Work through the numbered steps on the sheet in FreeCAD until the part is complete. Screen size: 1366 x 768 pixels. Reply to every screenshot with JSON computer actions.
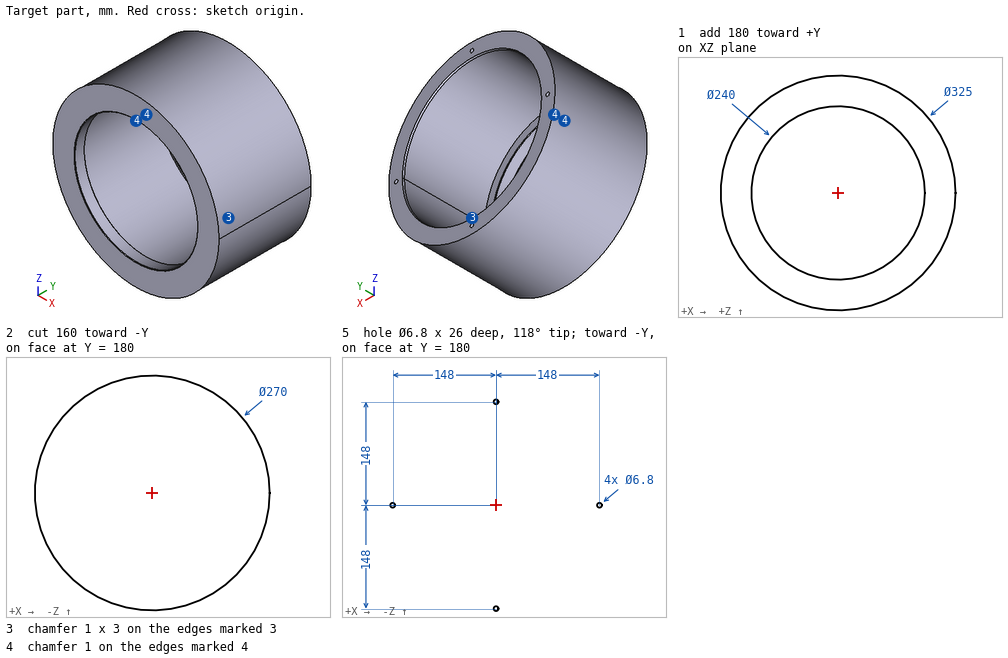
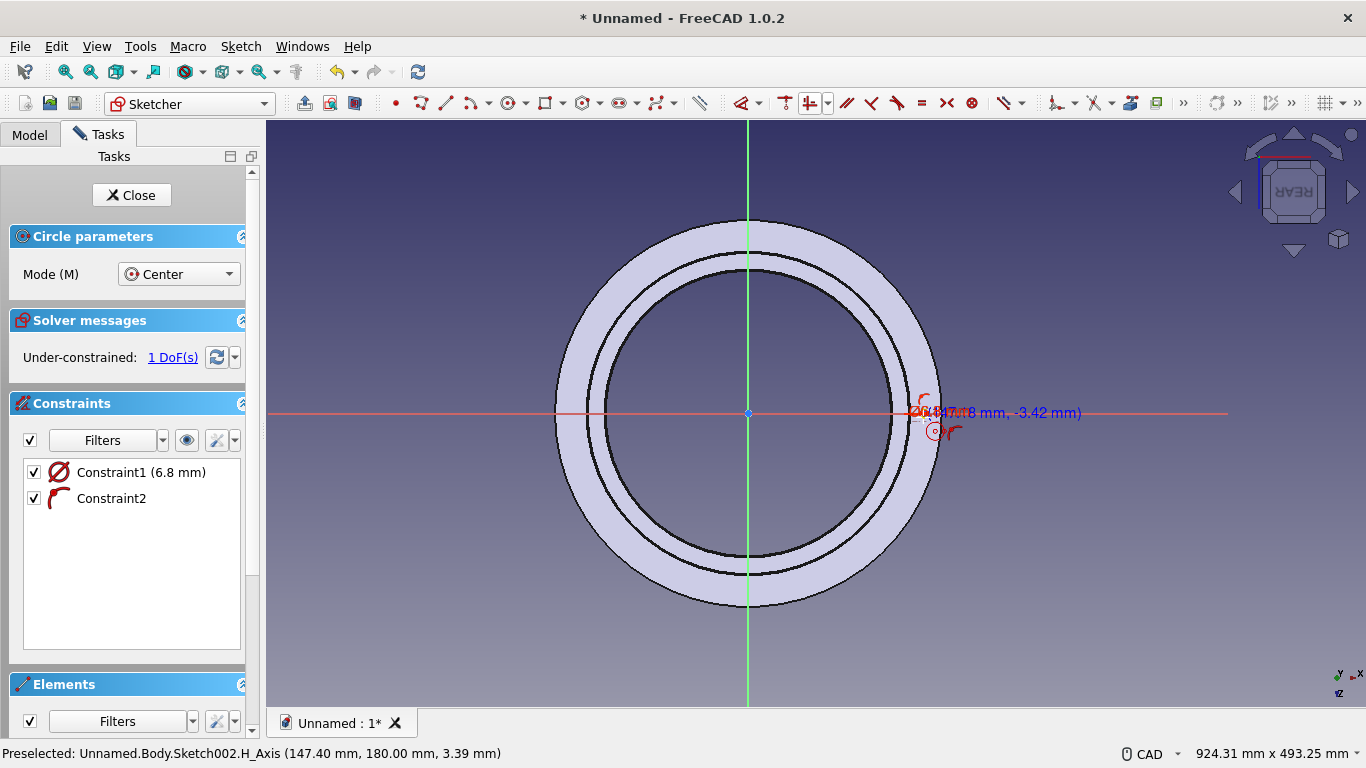
{"action": "scroll", "coordinate": [748, 590], "scroll_direction": "up", "scroll_amount": 9}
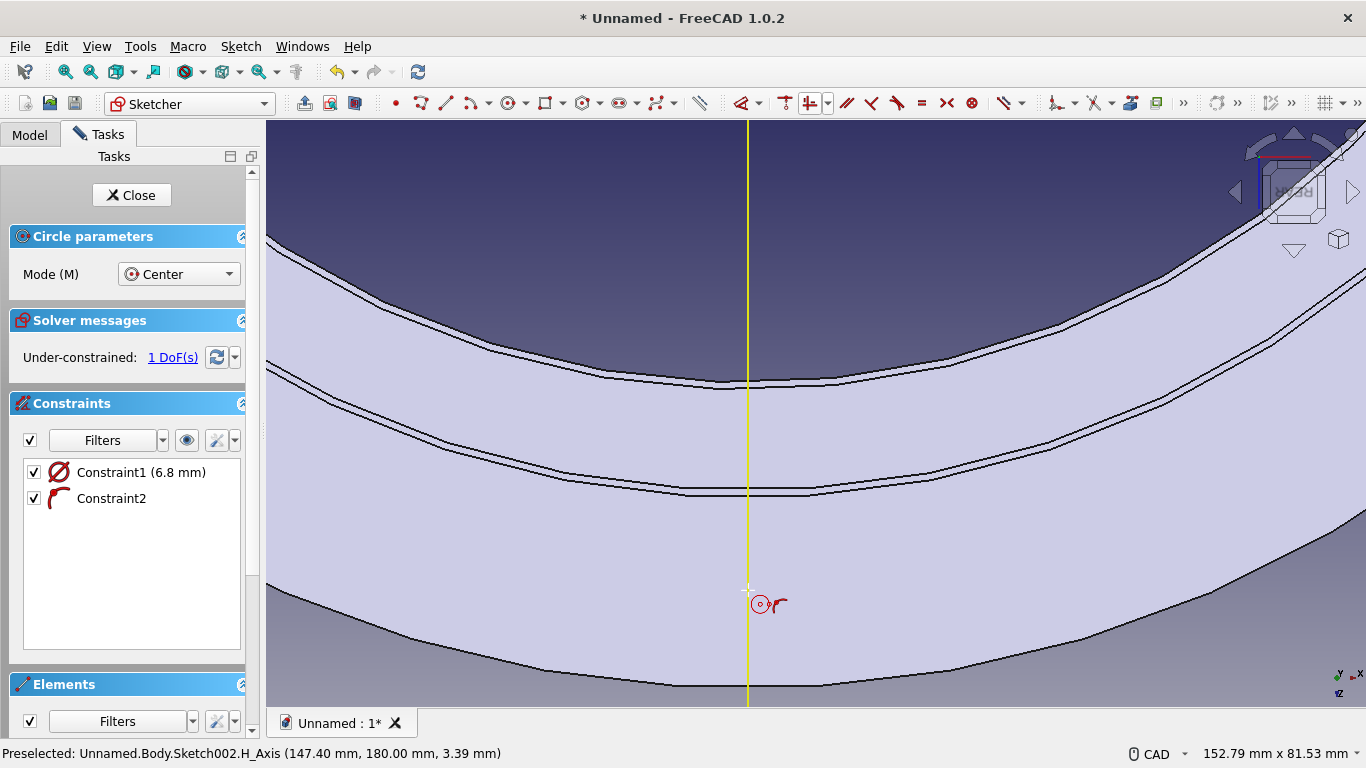
{"action": "scroll", "coordinate": [747, 591], "scroll_direction": "down", "scroll_amount": 9}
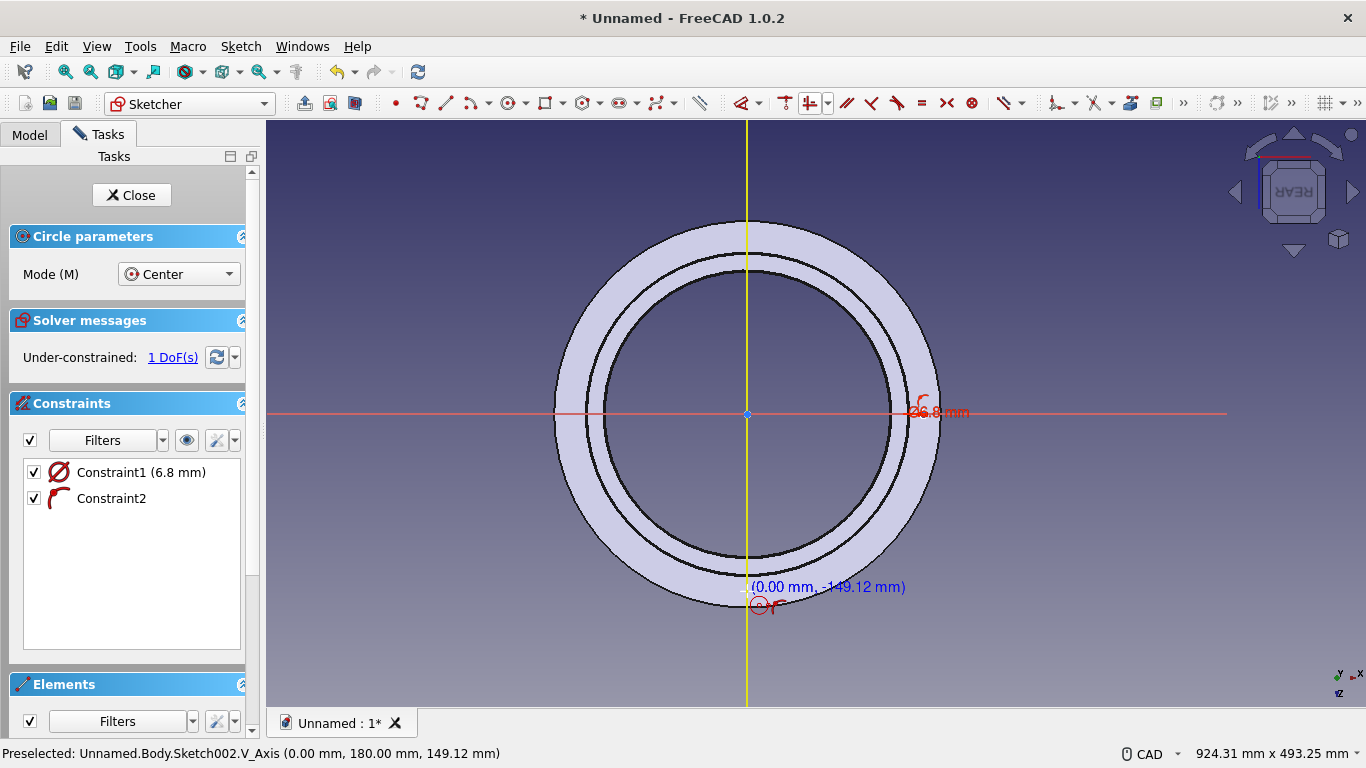
{"action": "left_click", "coordinate": [747, 591]}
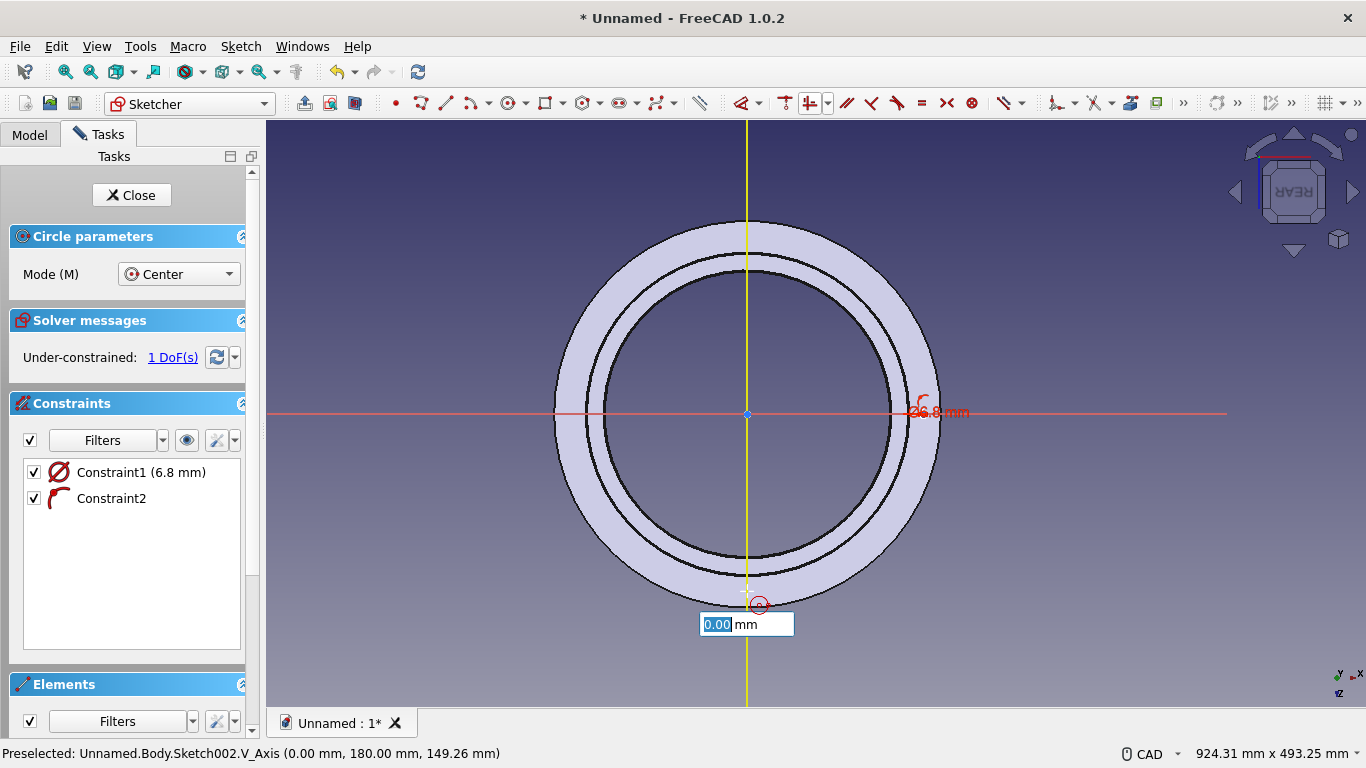
{"action": "scroll", "coordinate": [751, 589], "scroll_direction": "up", "scroll_amount": 8}
{"action": "mouse_move", "coordinate": [751, 586]}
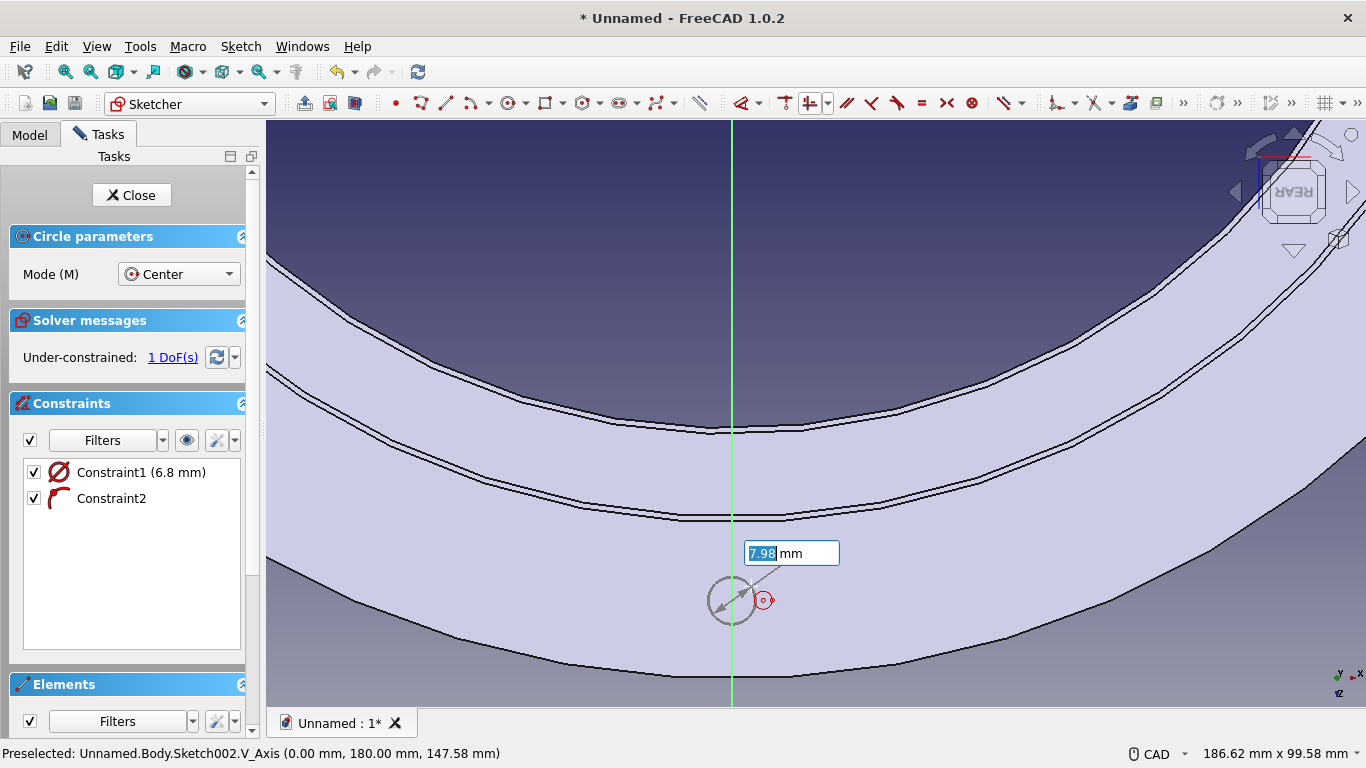
{"action": "type", "text": "6.8"}
{"action": "key", "text": "Return"}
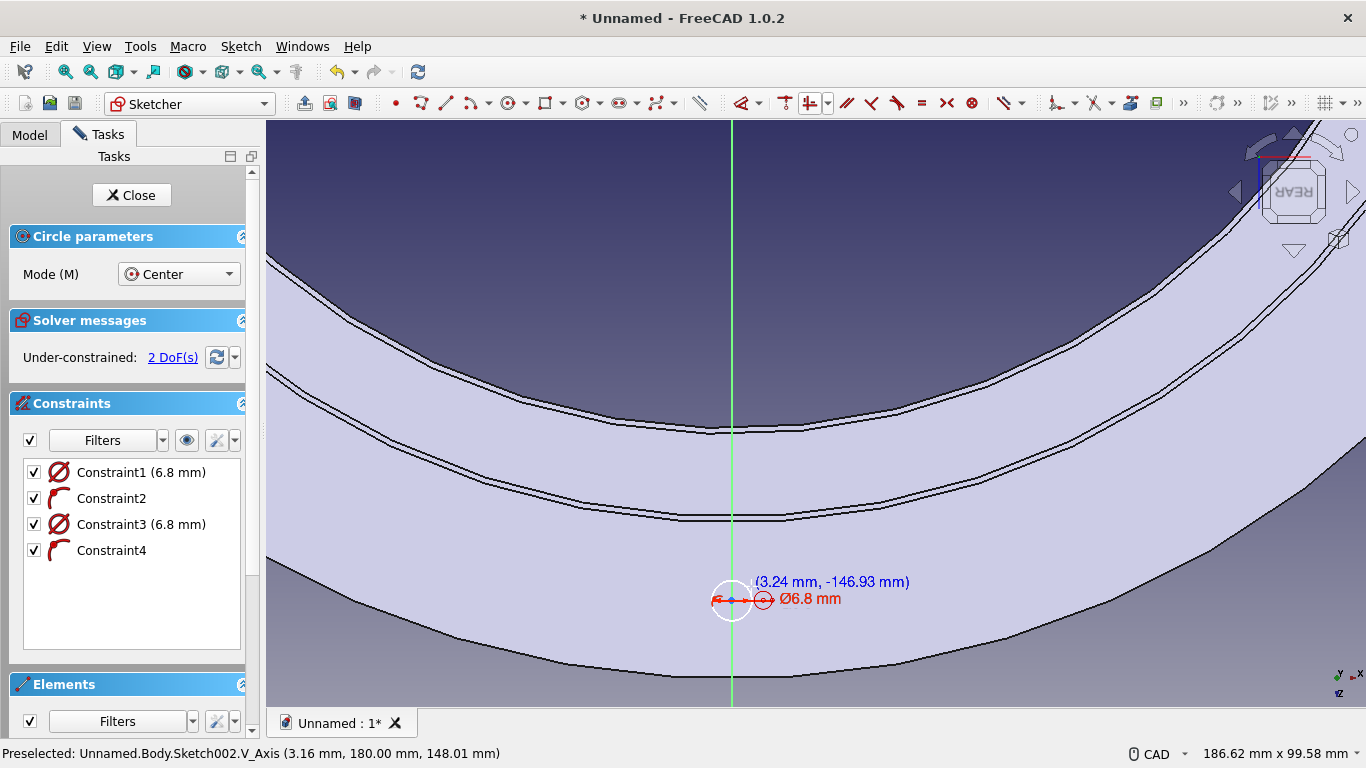
{"action": "scroll", "coordinate": [751, 589], "scroll_direction": "down", "scroll_amount": 8}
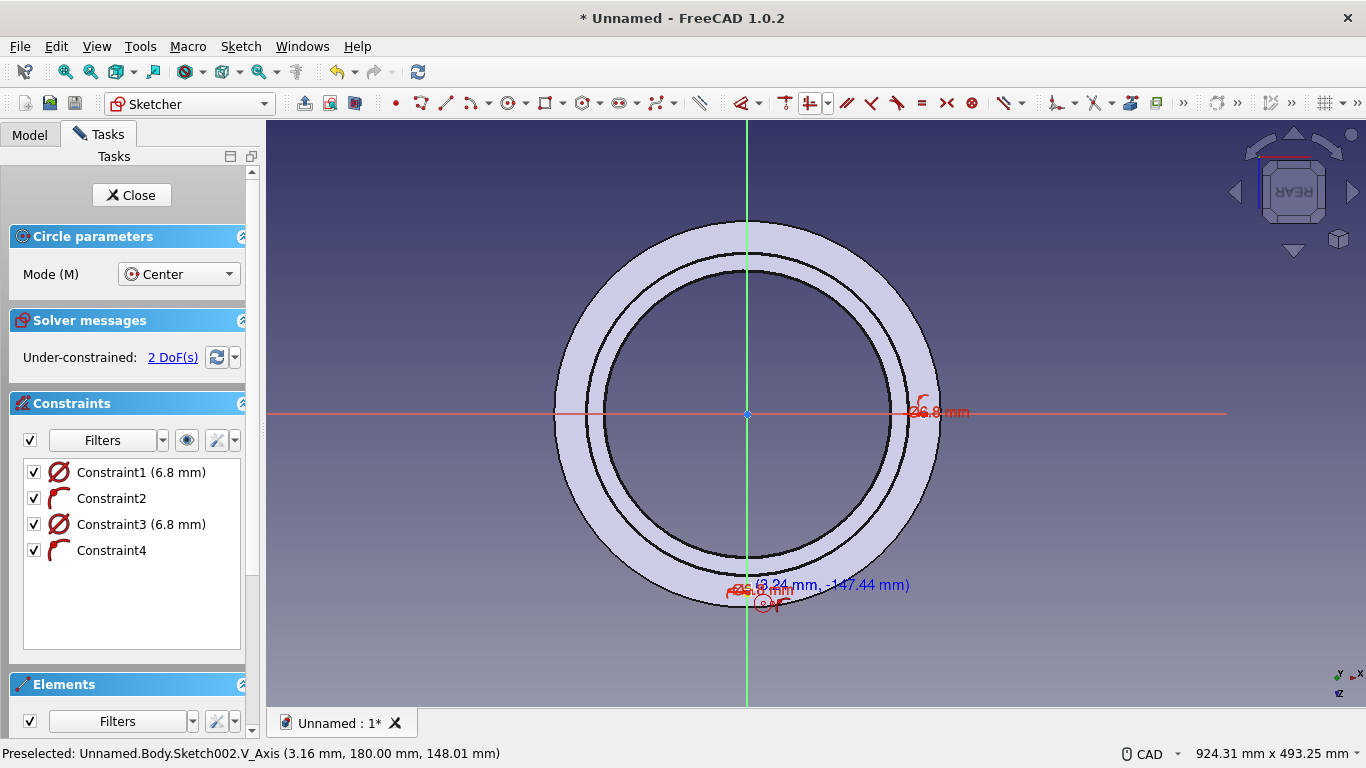
{"action": "scroll", "coordinate": [571, 414], "scroll_direction": "up", "scroll_amount": 9}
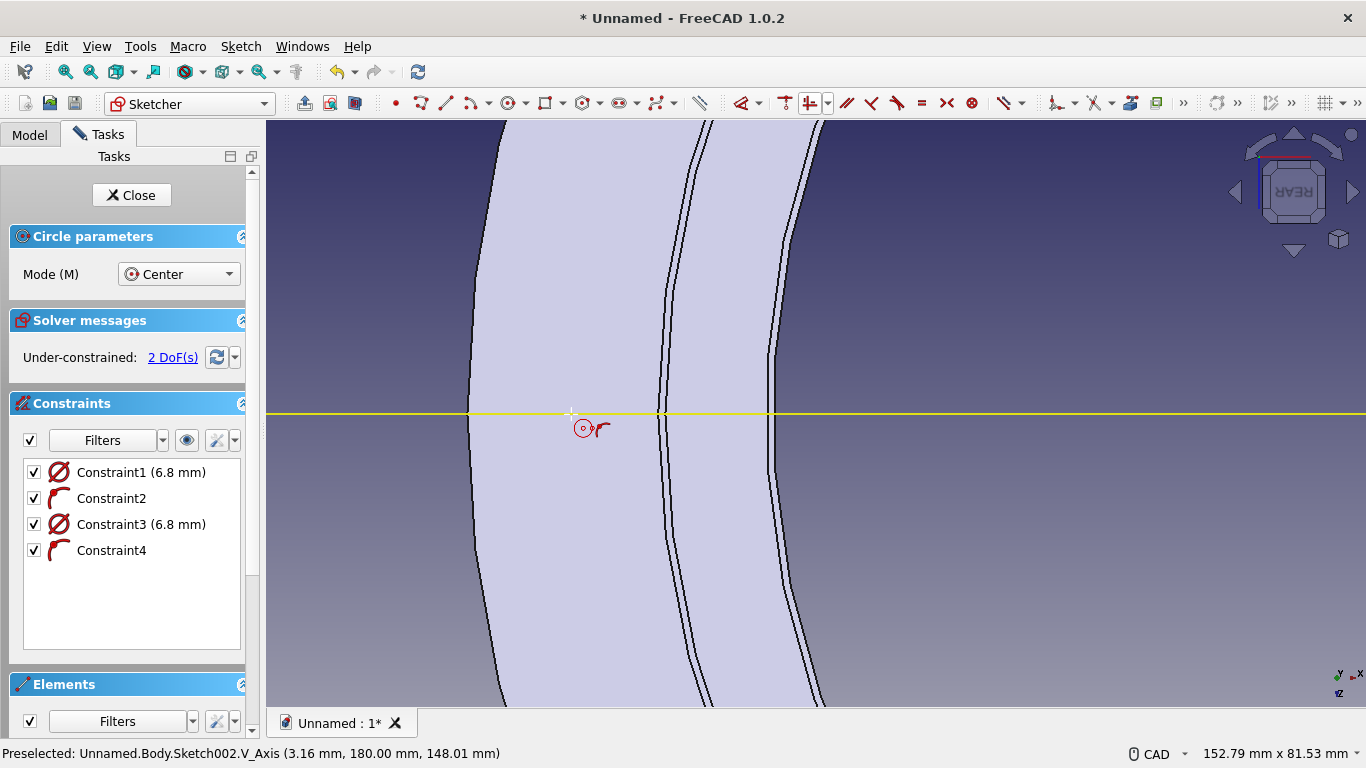
{"action": "scroll", "coordinate": [571, 413], "scroll_direction": "down", "scroll_amount": 9}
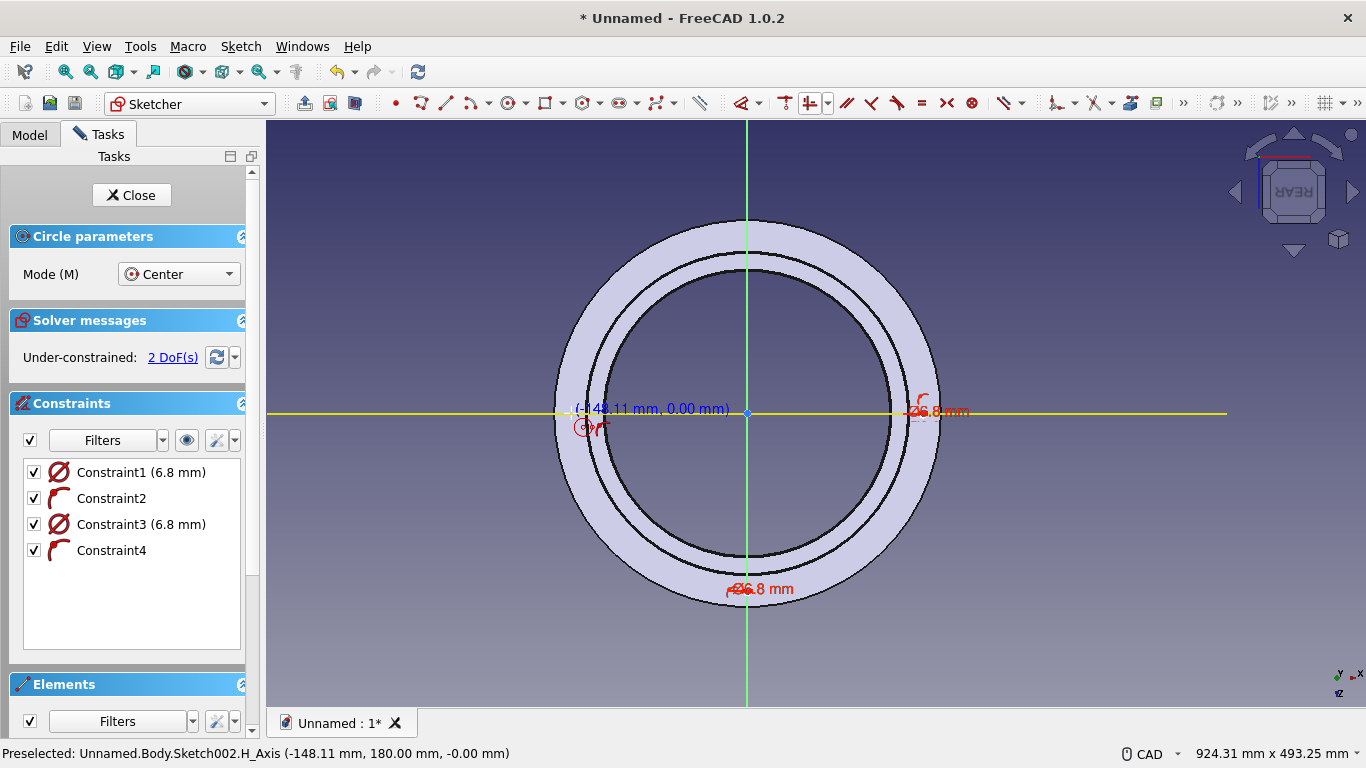
{"action": "left_click", "coordinate": [571, 414]}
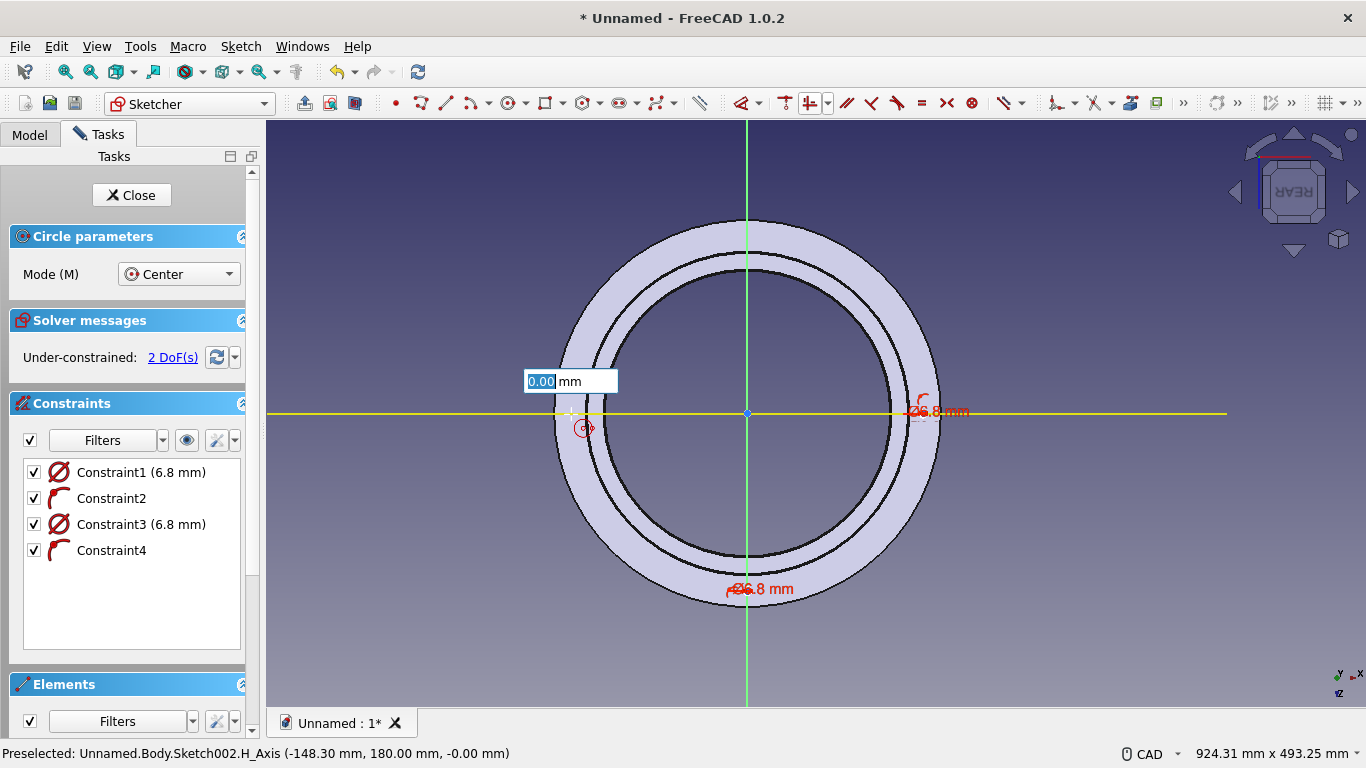
{"action": "scroll", "coordinate": [570, 417], "scroll_direction": "up", "scroll_amount": 8}
{"action": "mouse_move", "coordinate": [569, 417]}